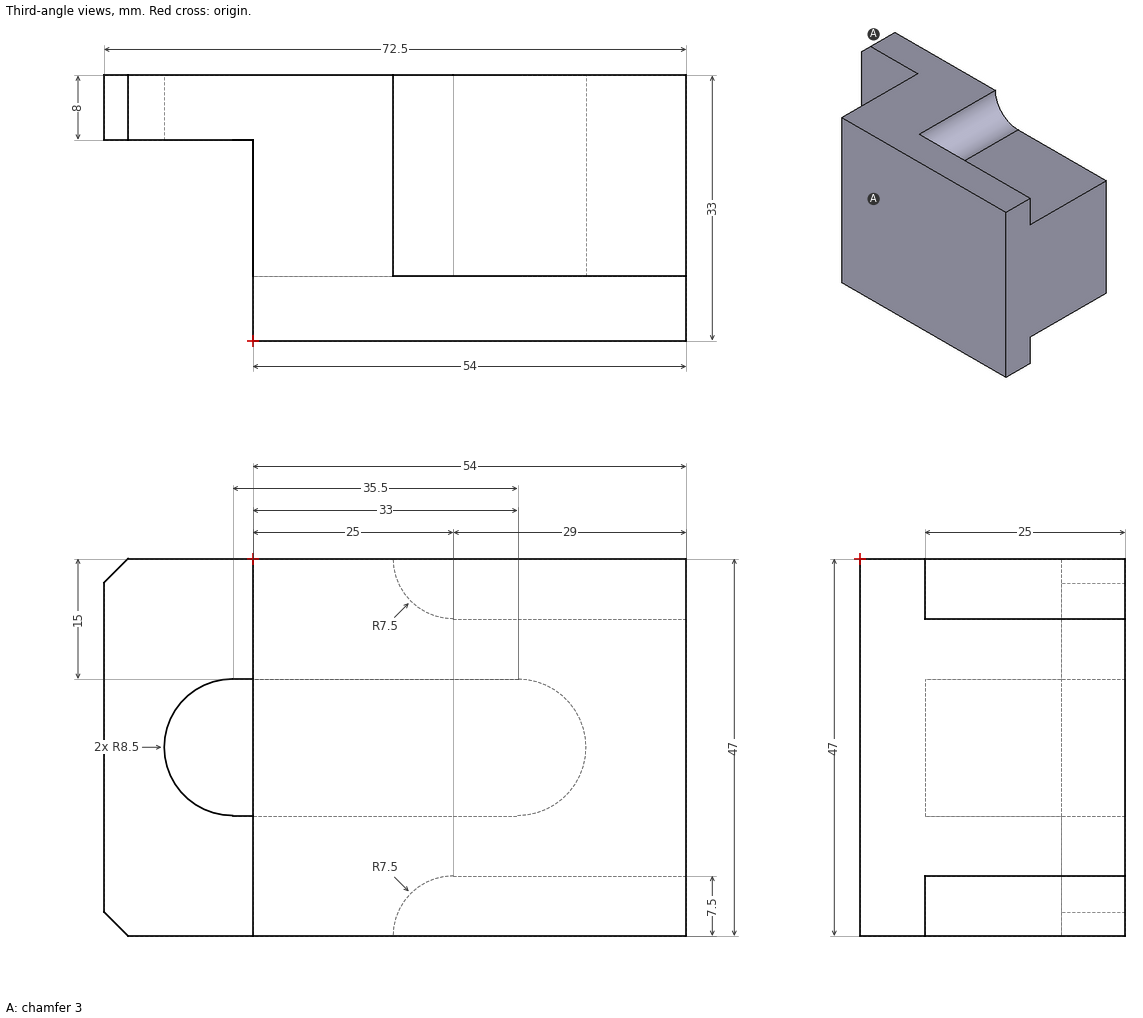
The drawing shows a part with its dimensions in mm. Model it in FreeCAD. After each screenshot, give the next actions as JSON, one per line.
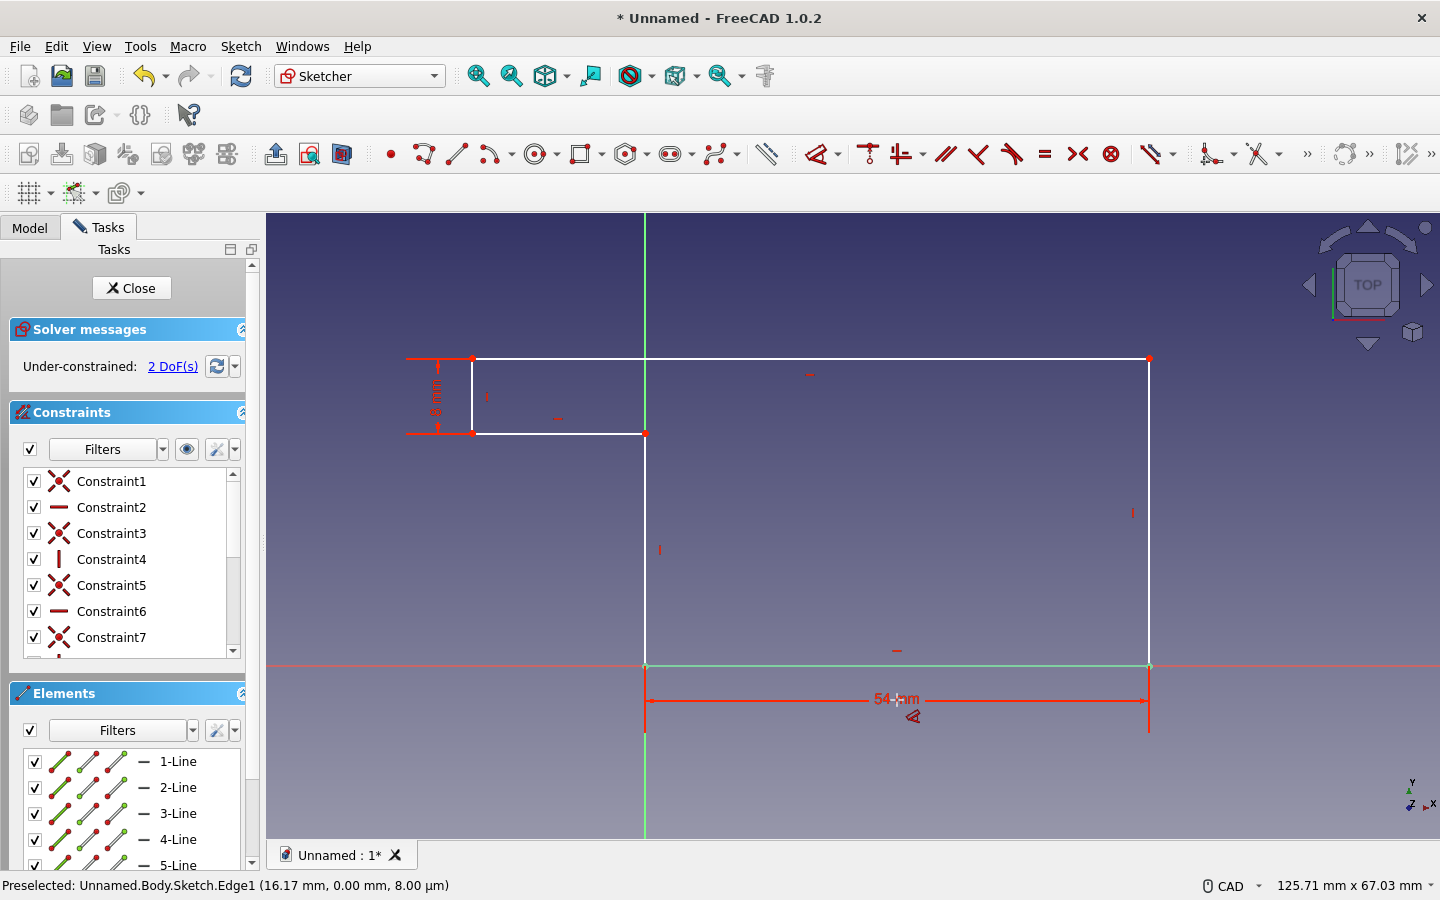
{"action": "left_click", "coordinate": [1149, 574]}
{"action": "left_click", "coordinate": [1183, 513]}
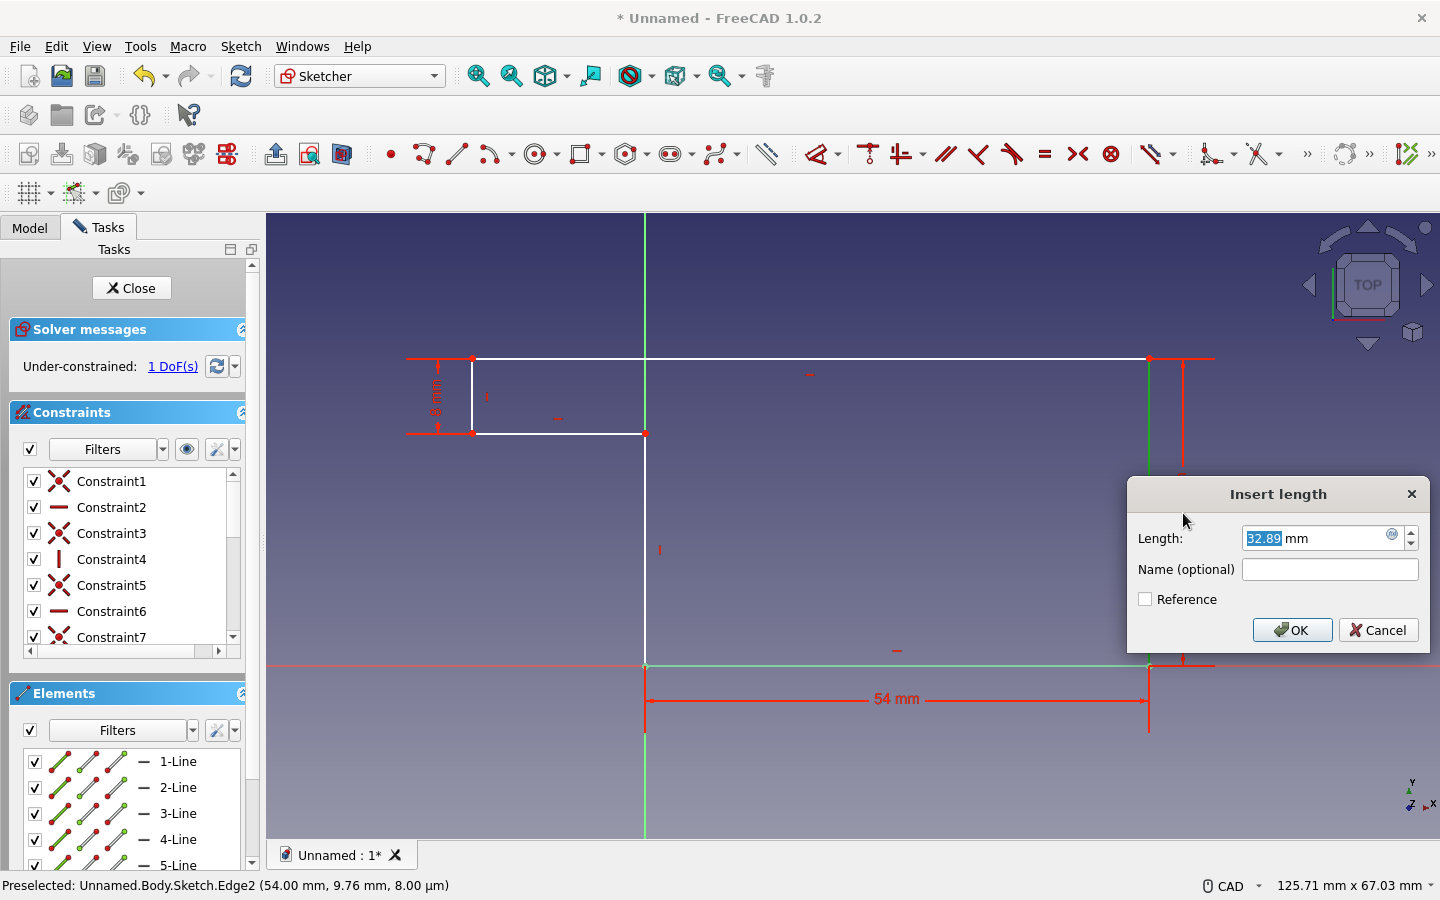
{"action": "type", "text": "33"}
{"action": "key", "text": "Return"}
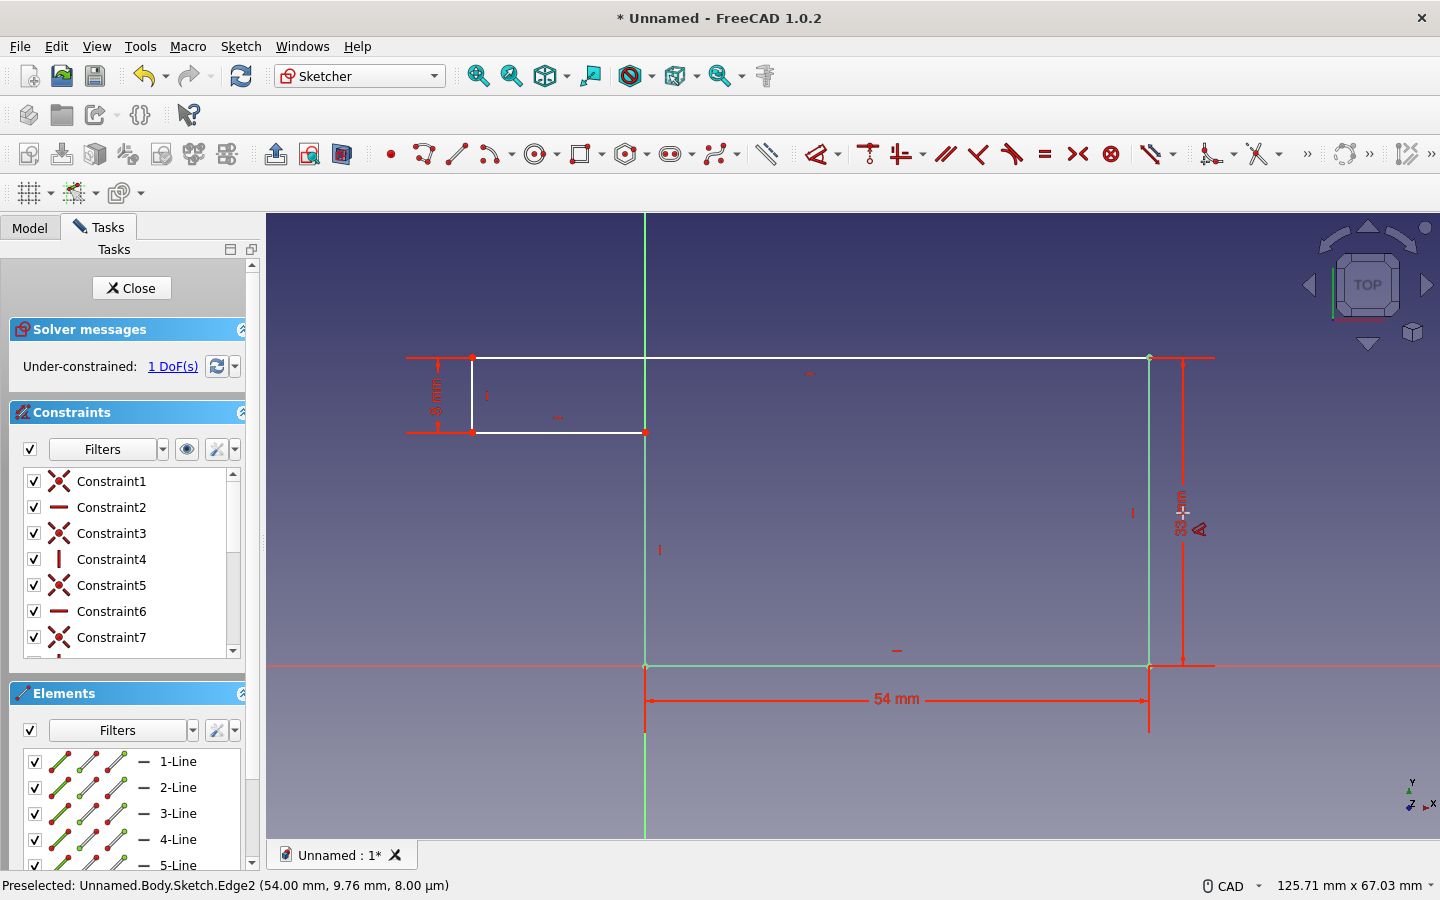
{"action": "left_click", "coordinate": [946, 358]}
{"action": "left_click", "coordinate": [811, 324]}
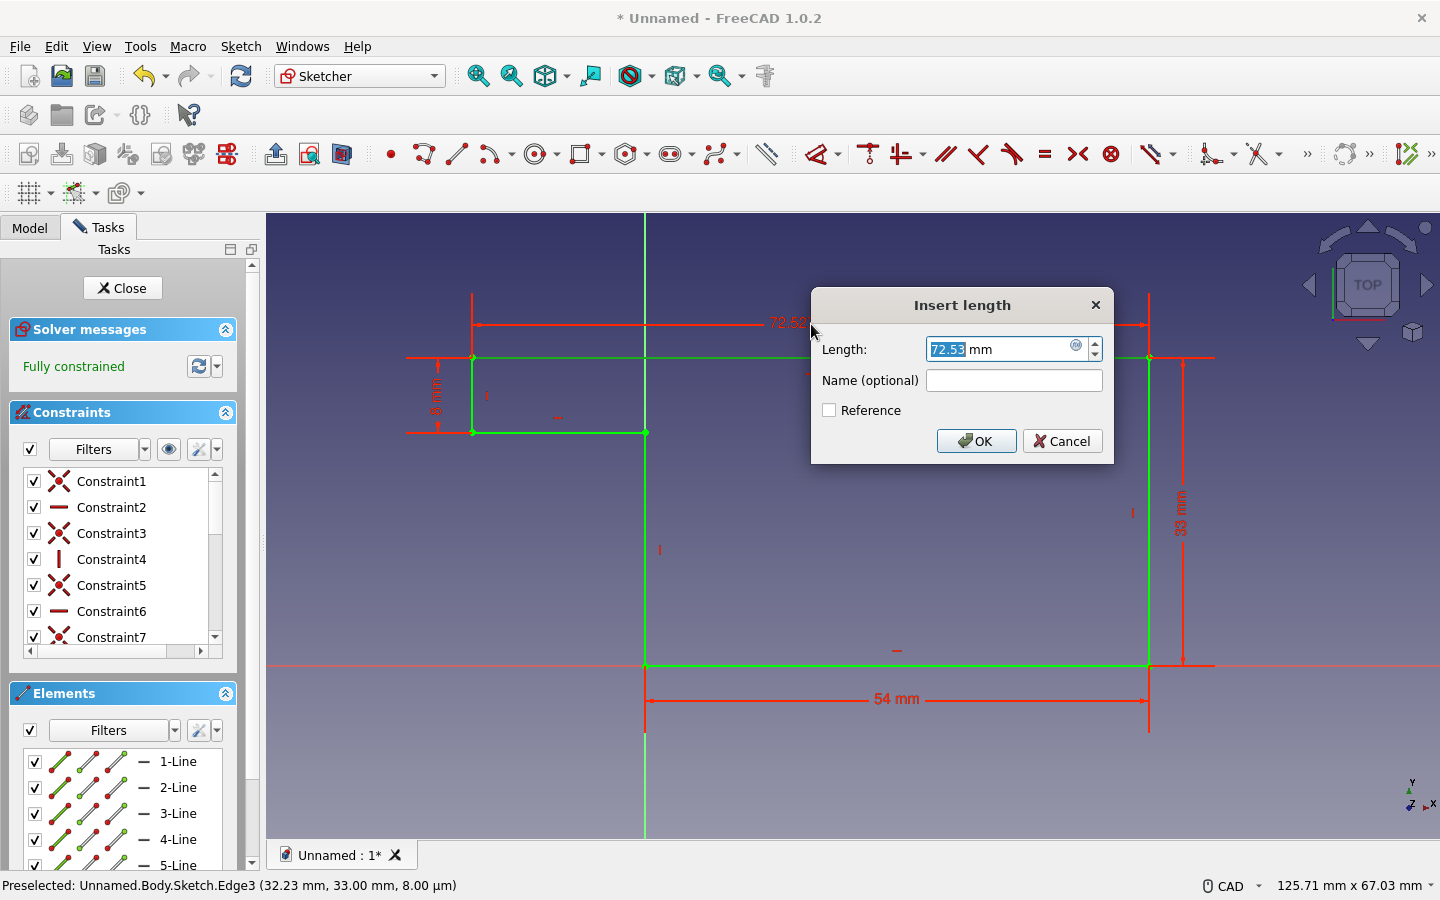
{"action": "type", "text": "72.5"}
{"action": "key", "text": "Return"}
{"action": "key", "text": "Escape"}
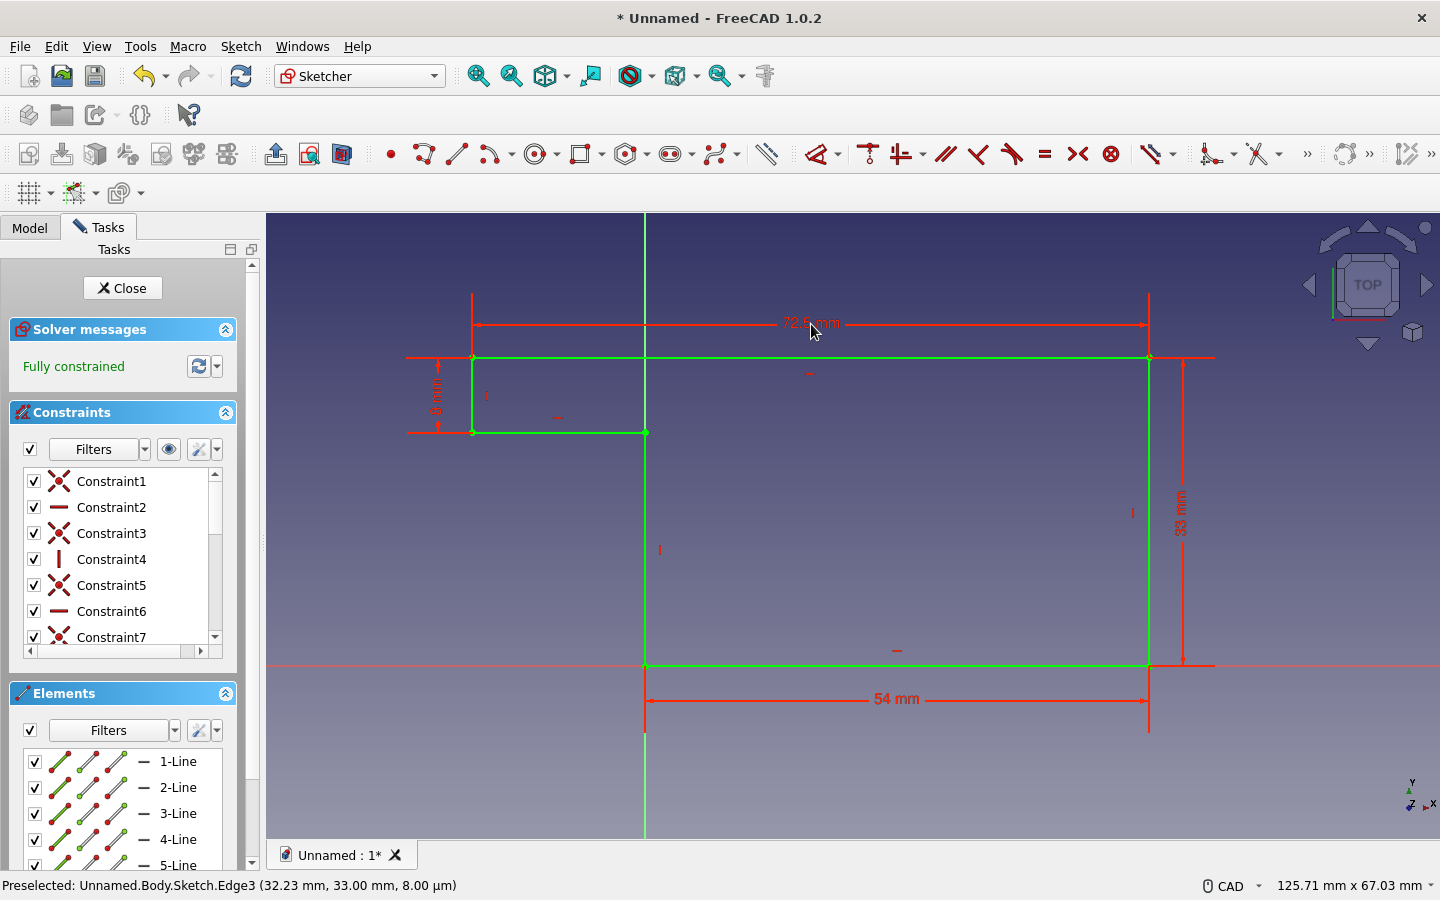
{"action": "left_click", "coordinate": [123, 288]}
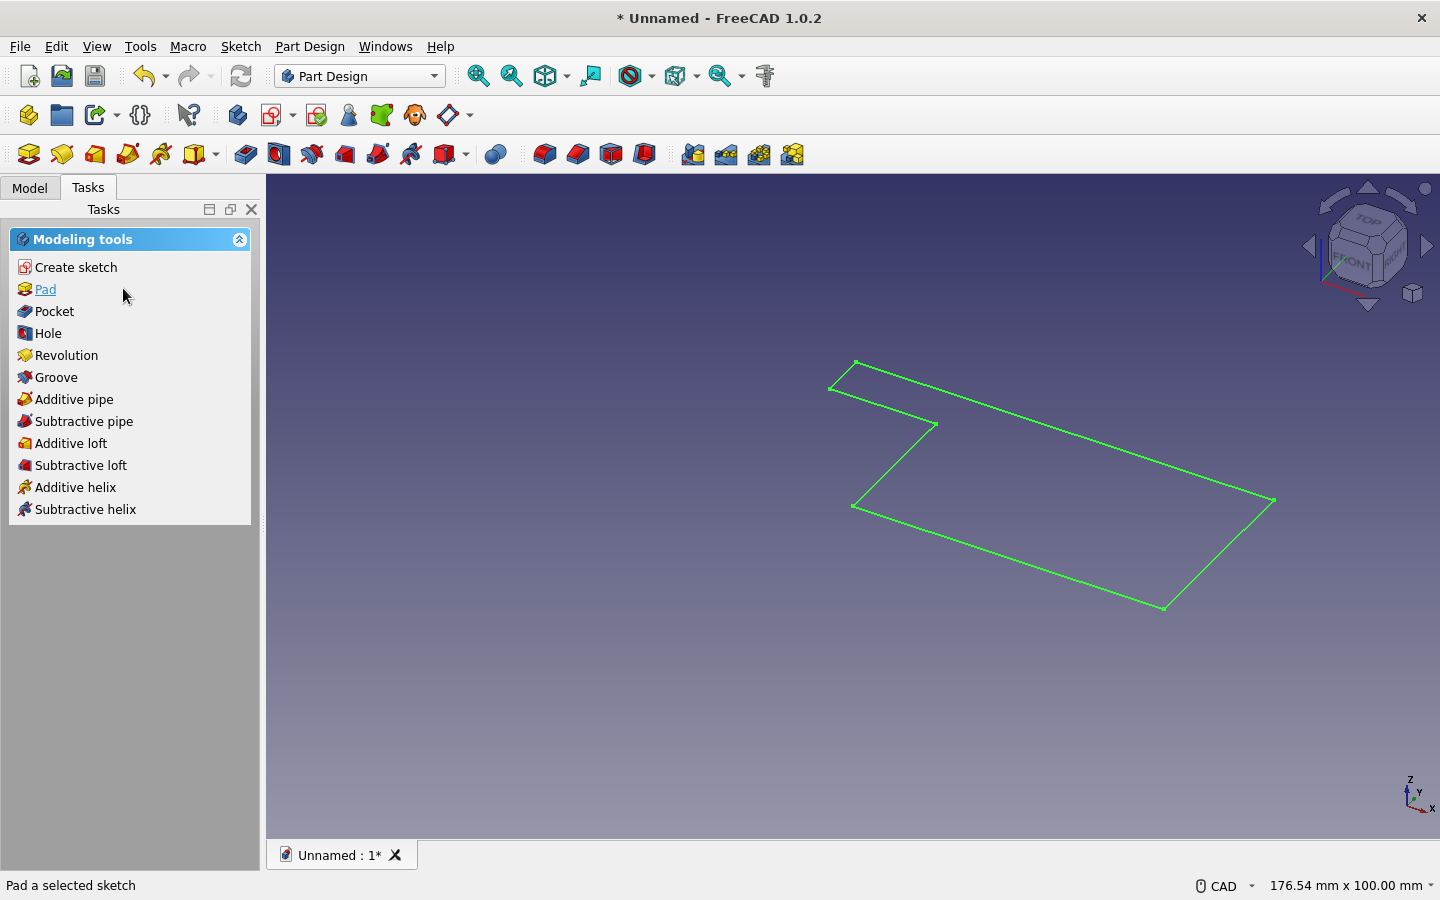
{"action": "left_click", "coordinate": [29, 154]}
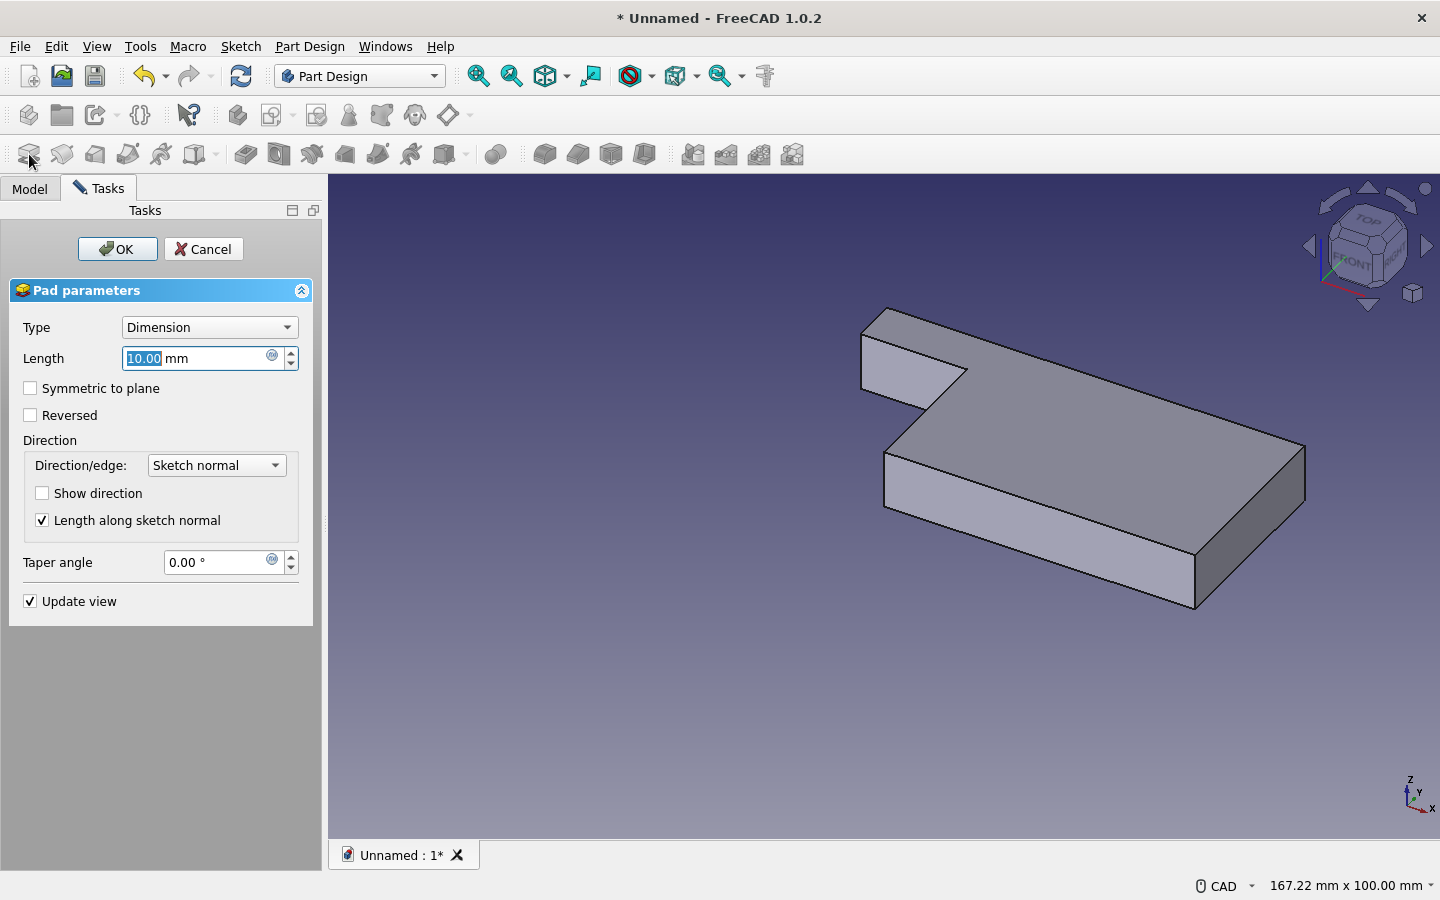
{"action": "type", "text": "47"}
{"action": "key", "text": "Tab"}